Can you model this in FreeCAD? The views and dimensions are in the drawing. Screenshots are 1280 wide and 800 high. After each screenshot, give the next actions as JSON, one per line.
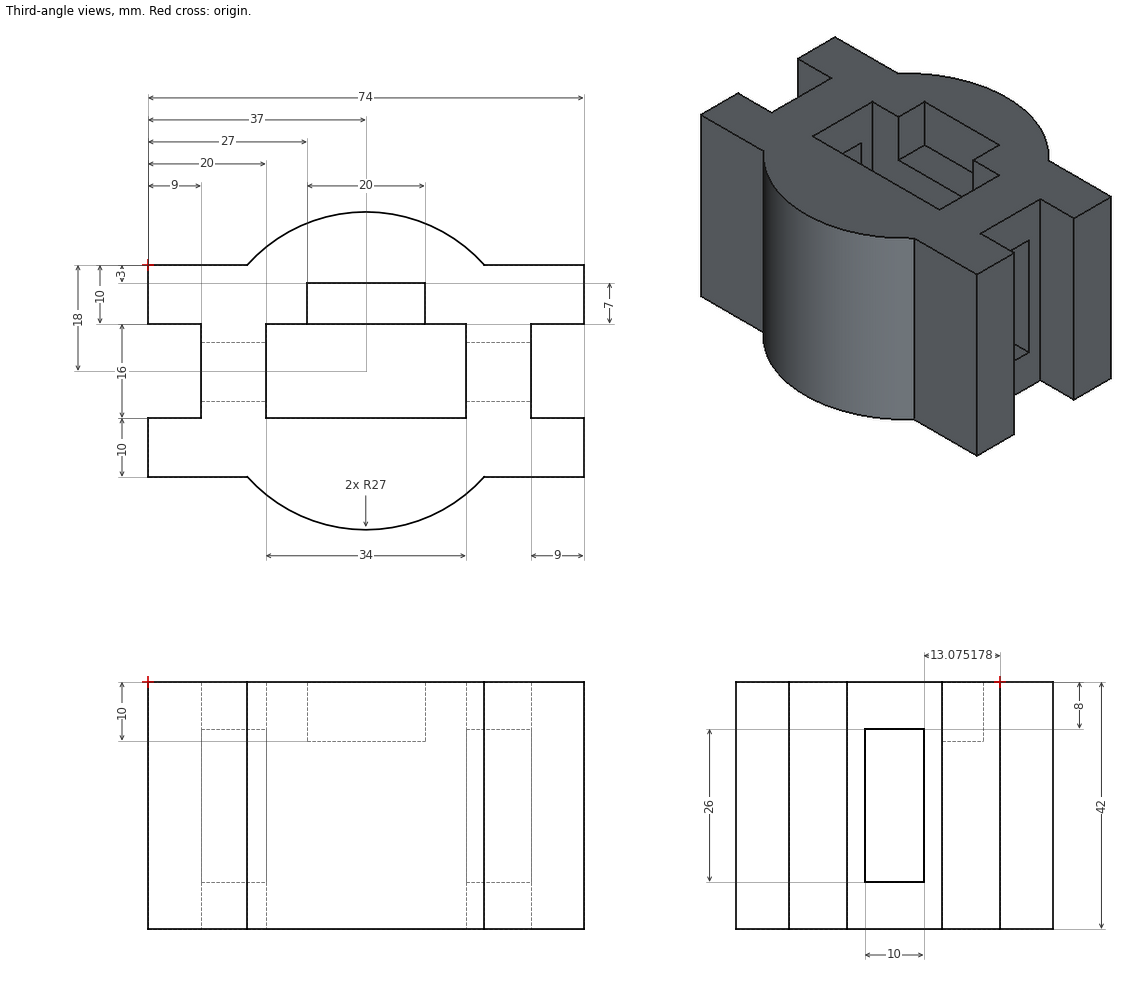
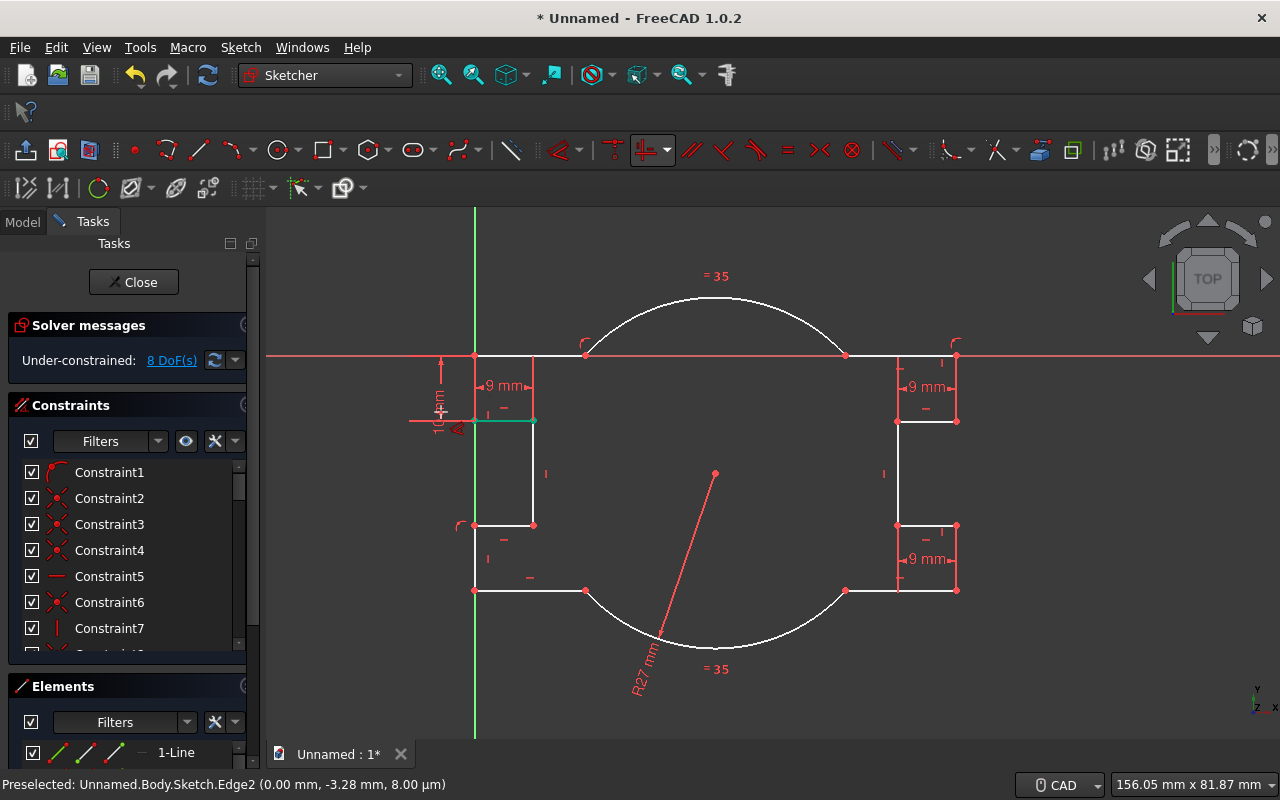
{"action": "left_click", "coordinate": [533, 452]}
{"action": "left_click", "coordinate": [499, 473]}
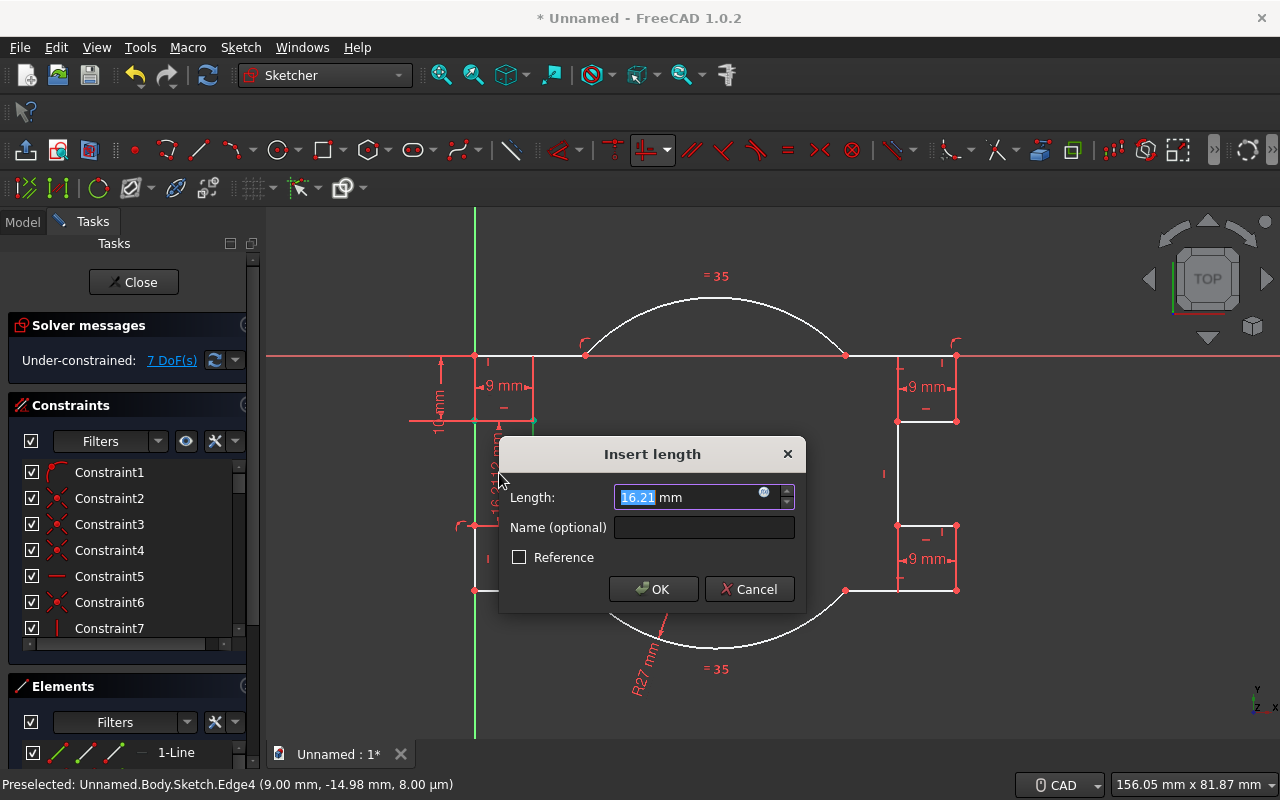
{"action": "type", "text": "16"}
{"action": "key", "text": "Return"}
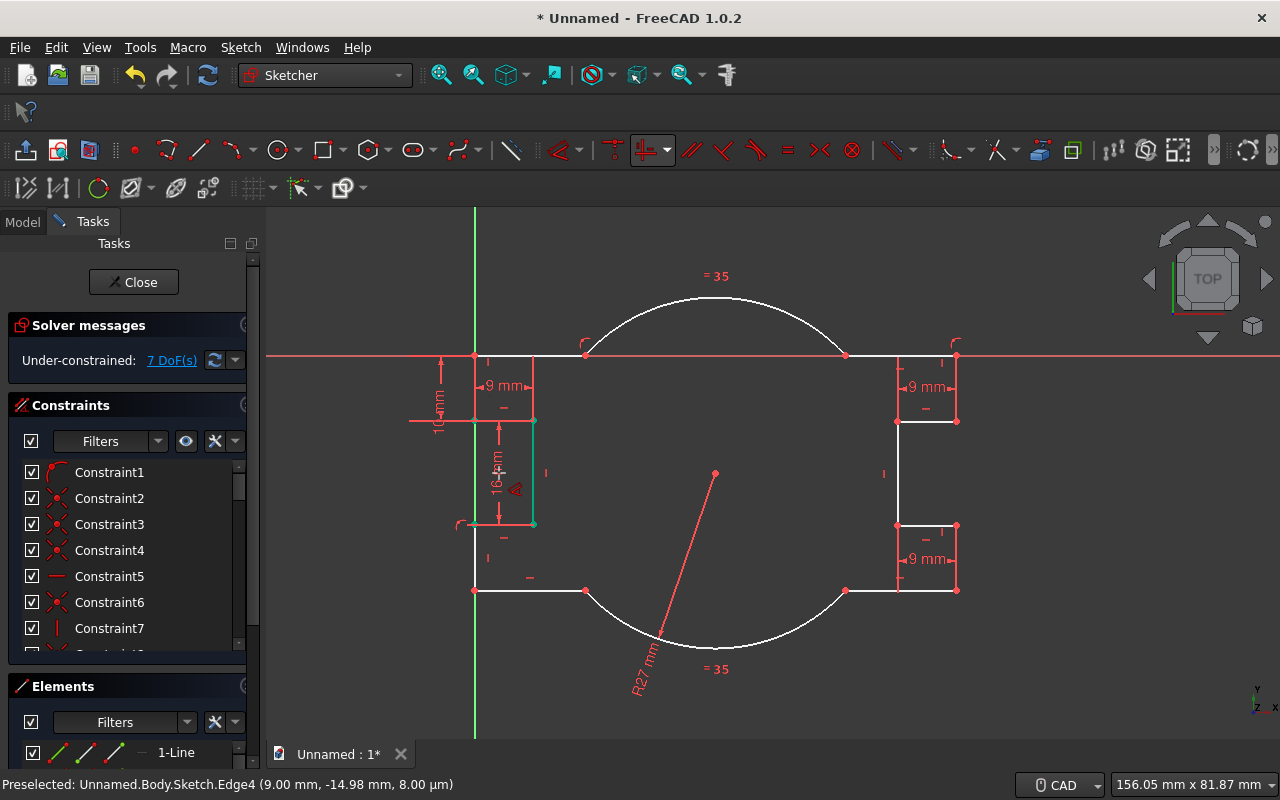
{"action": "left_click", "coordinate": [475, 544]}
{"action": "left_click", "coordinate": [441, 558]}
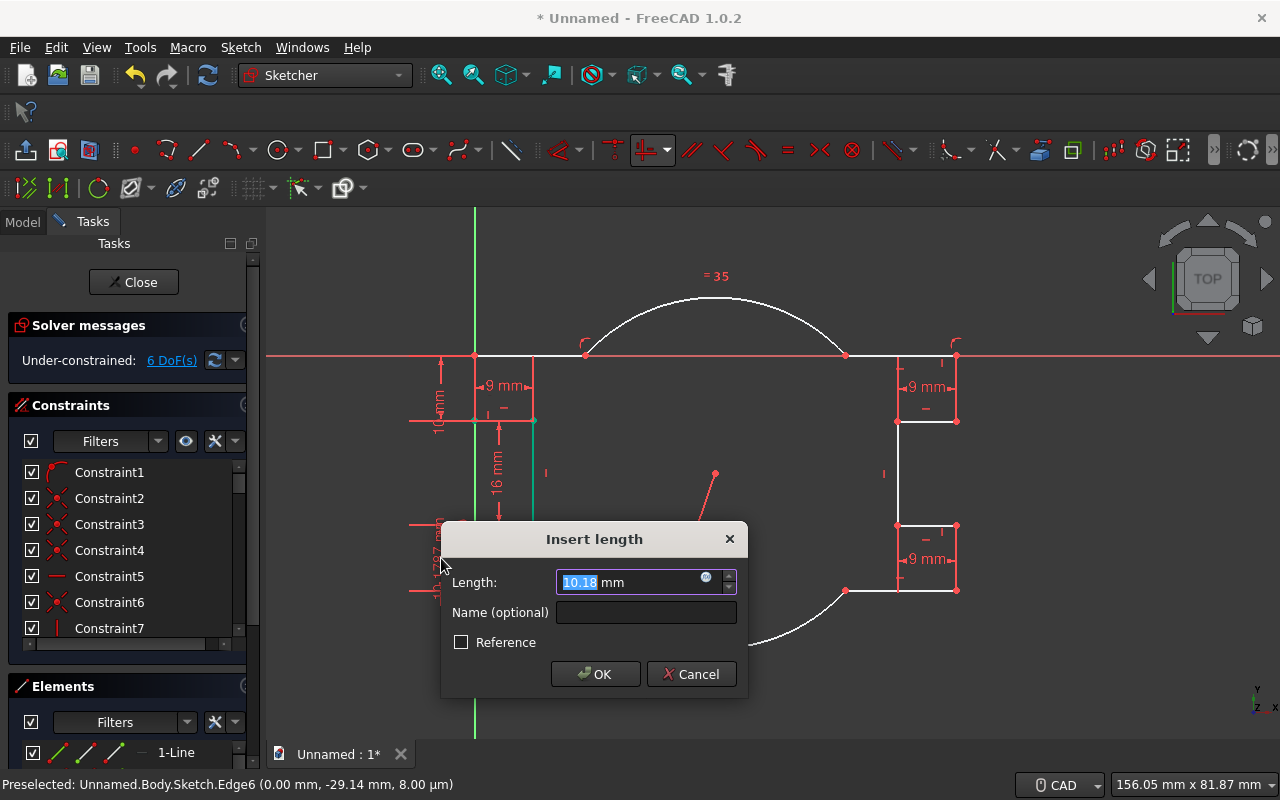
{"action": "type", "text": "10"}
{"action": "key", "text": "Return"}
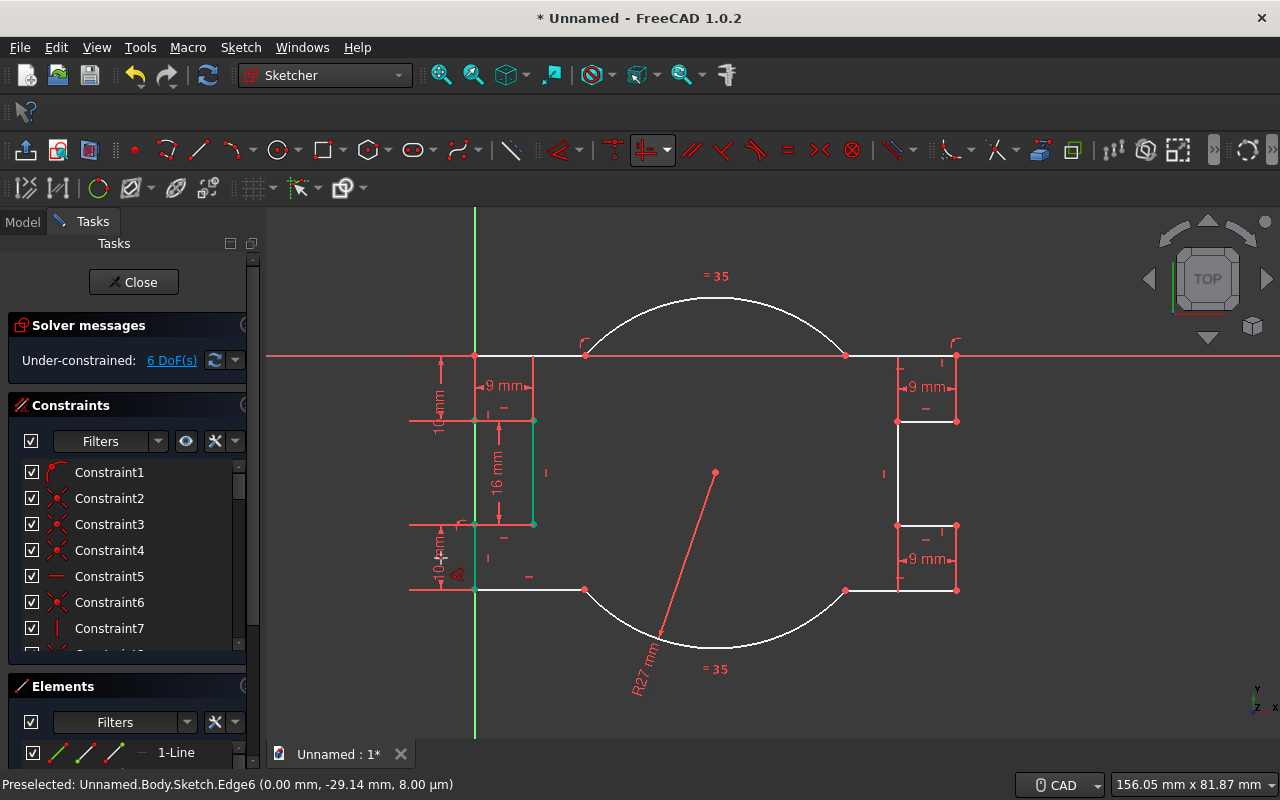
{"action": "left_click", "coordinate": [956, 571]}
{"action": "left_click", "coordinate": [990, 536]}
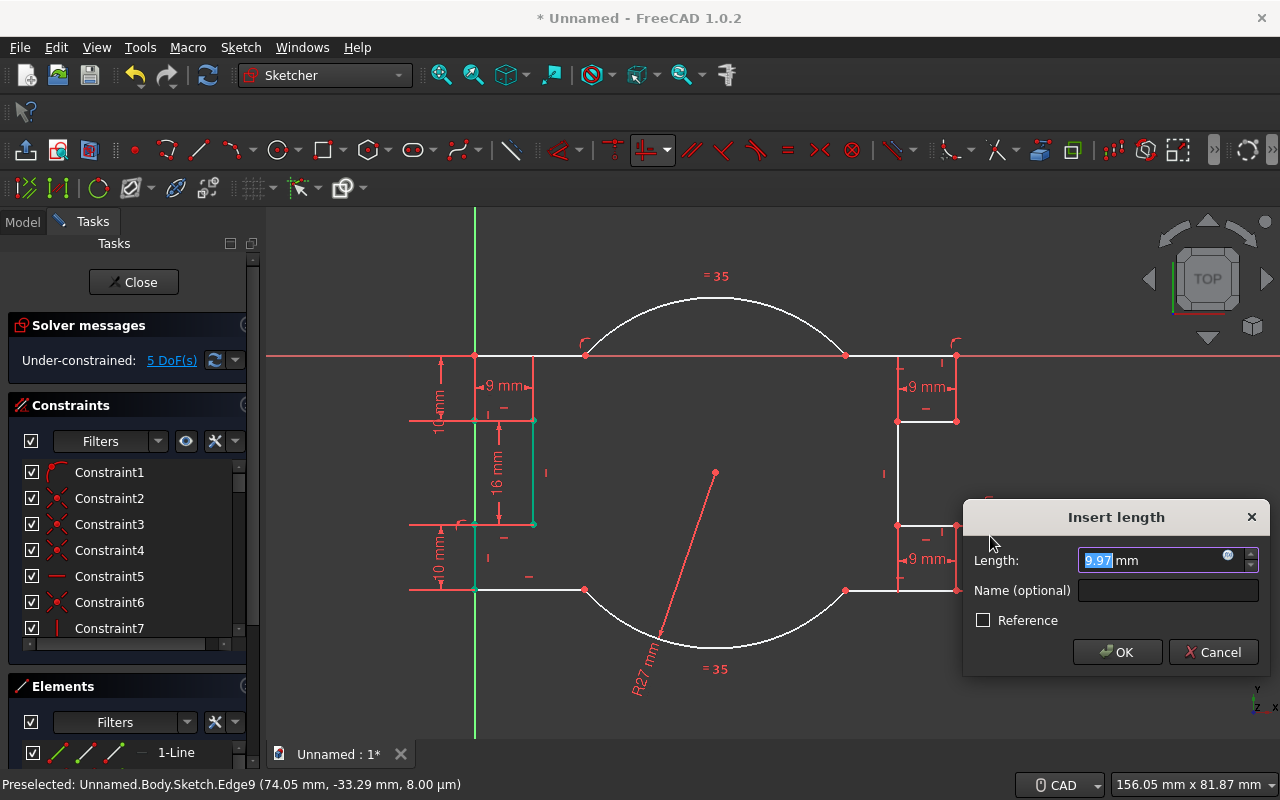
{"action": "type", "text": "10"}
{"action": "key", "text": "Return"}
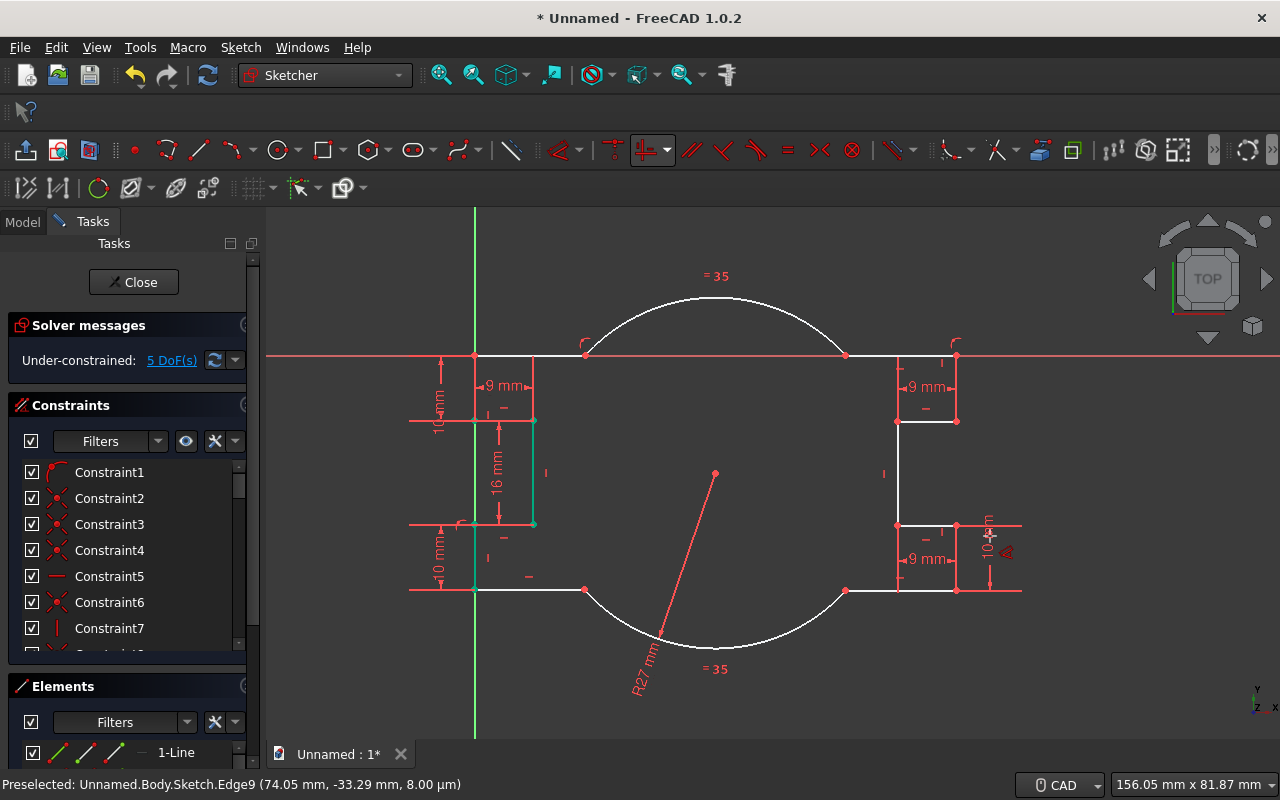
{"action": "left_click", "coordinate": [898, 495]}
{"action": "left_click", "coordinate": [932, 474]}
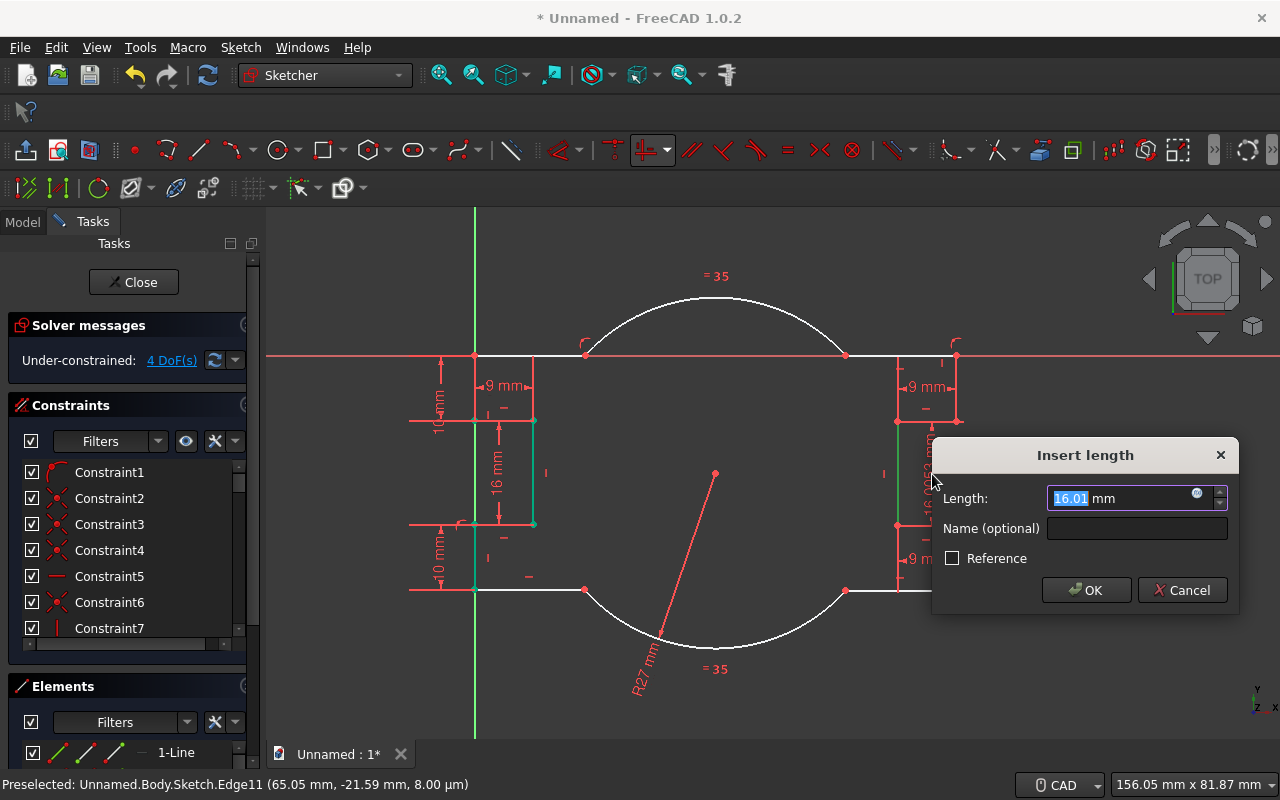
{"action": "type", "text": "16"}
{"action": "key", "text": "Return"}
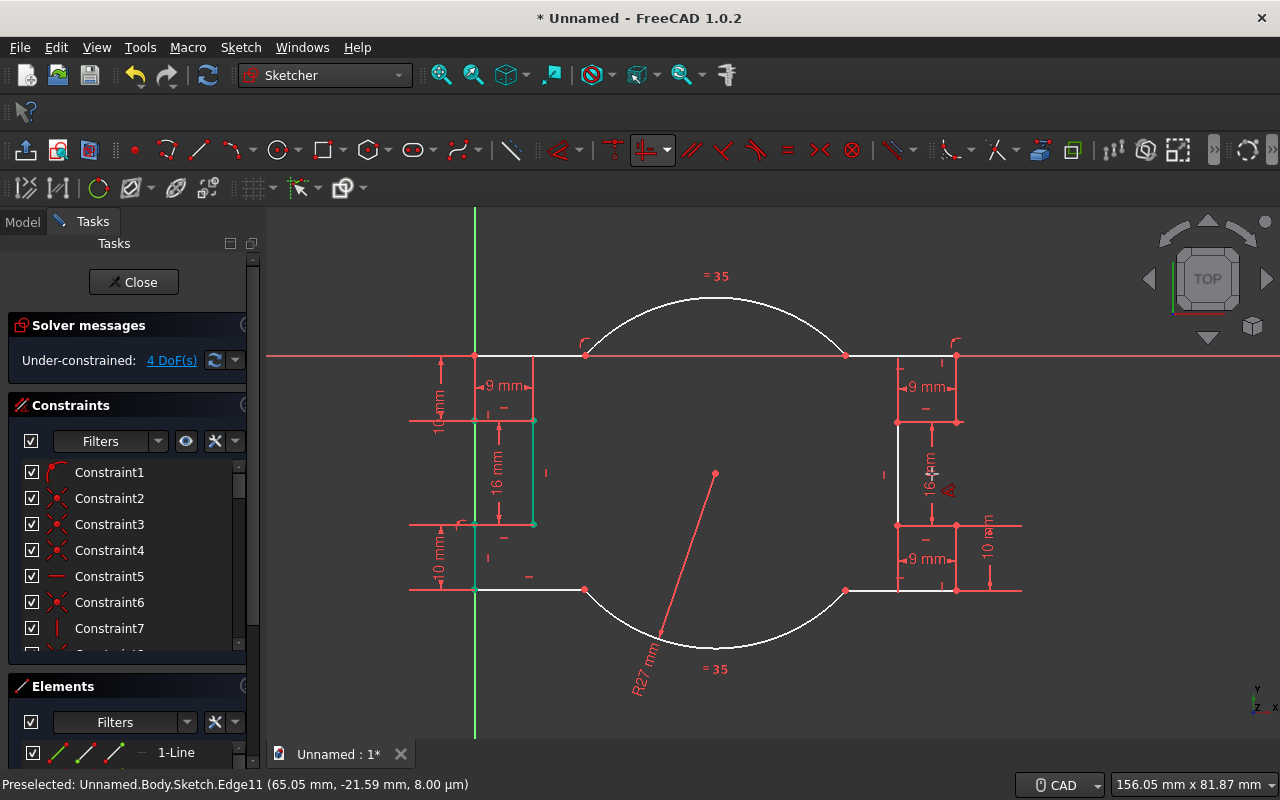
{"action": "left_click", "coordinate": [956, 402]}
{"action": "left_click", "coordinate": [990, 412]}